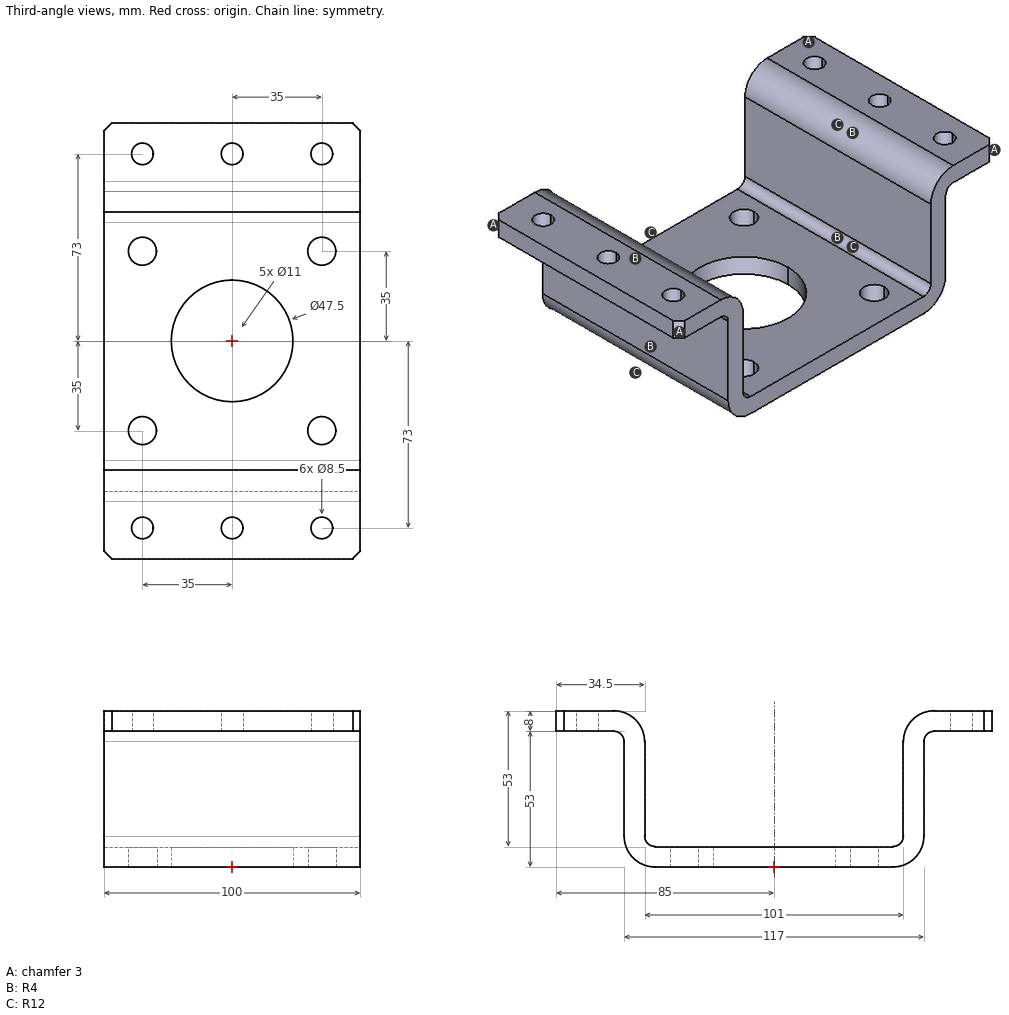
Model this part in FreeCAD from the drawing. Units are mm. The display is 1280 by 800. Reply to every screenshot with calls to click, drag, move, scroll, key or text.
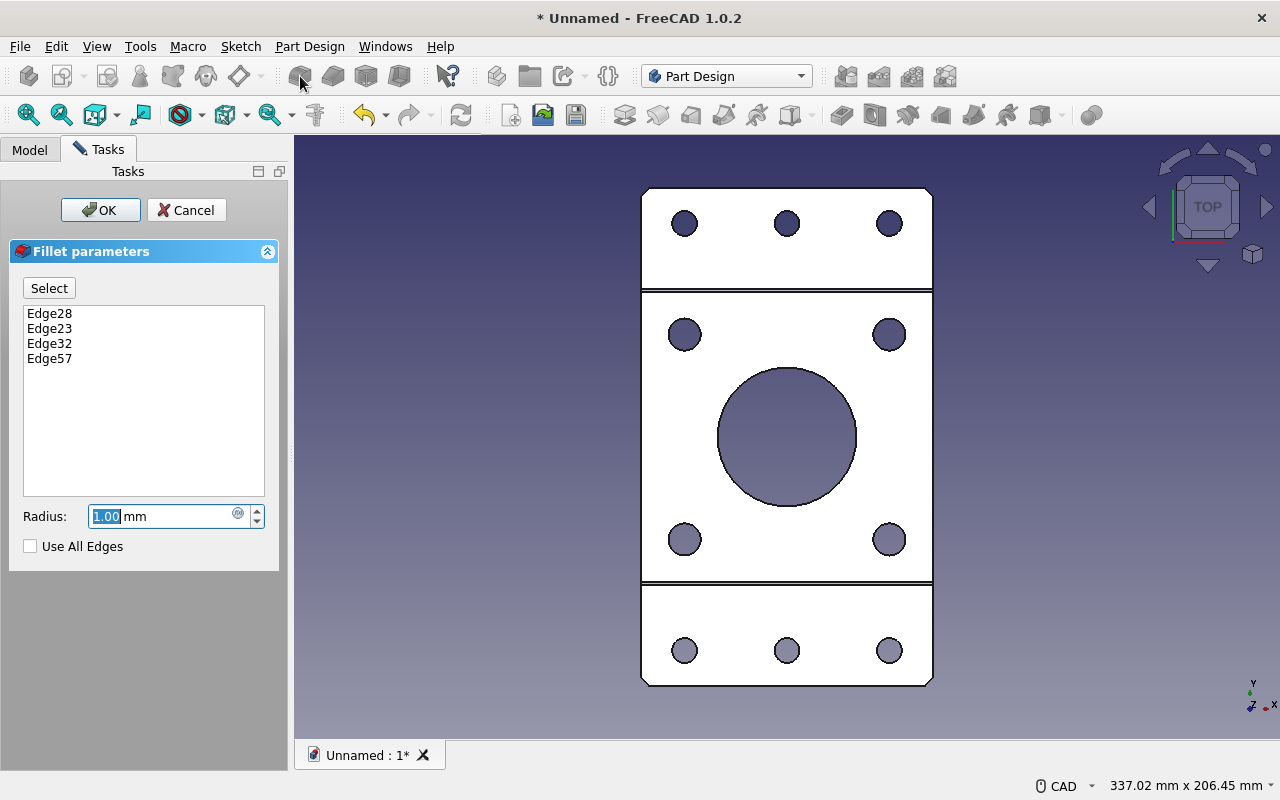
text(4)
key(Tab)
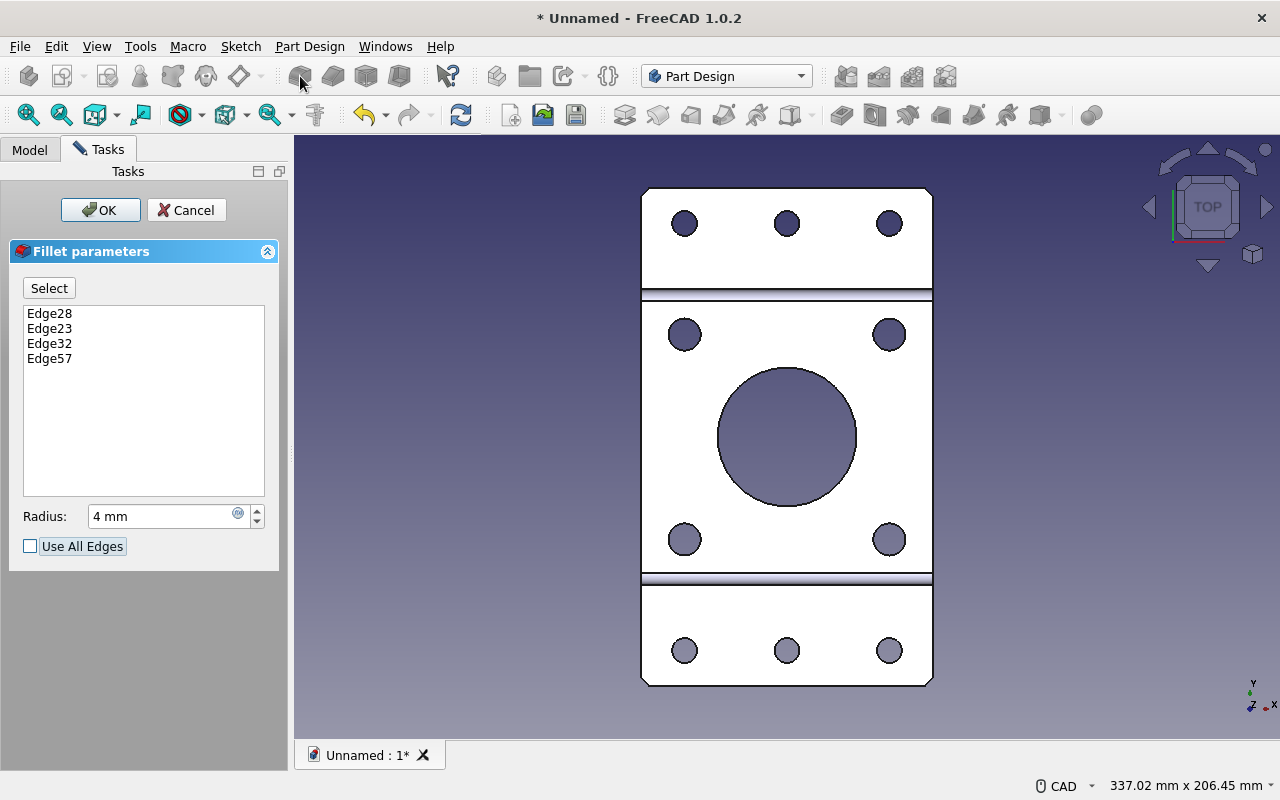
click(101, 210)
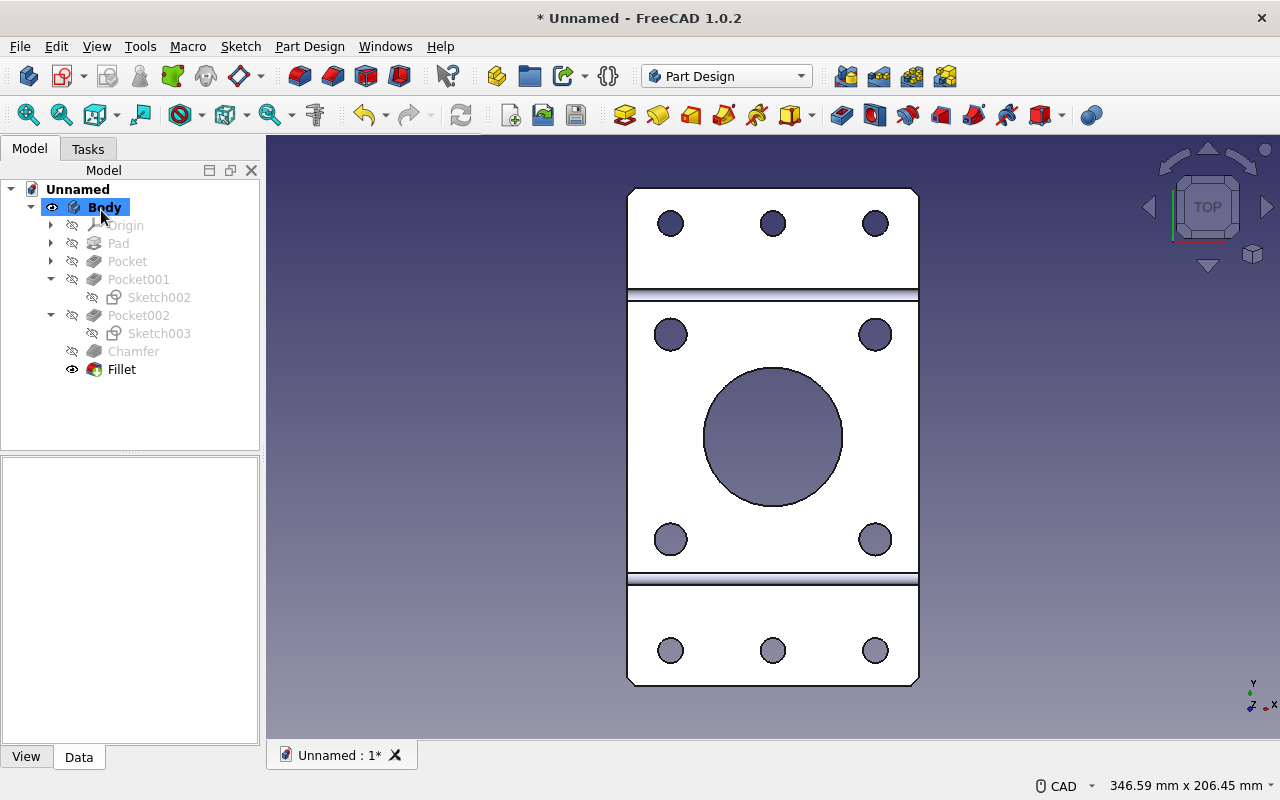
click(773, 584)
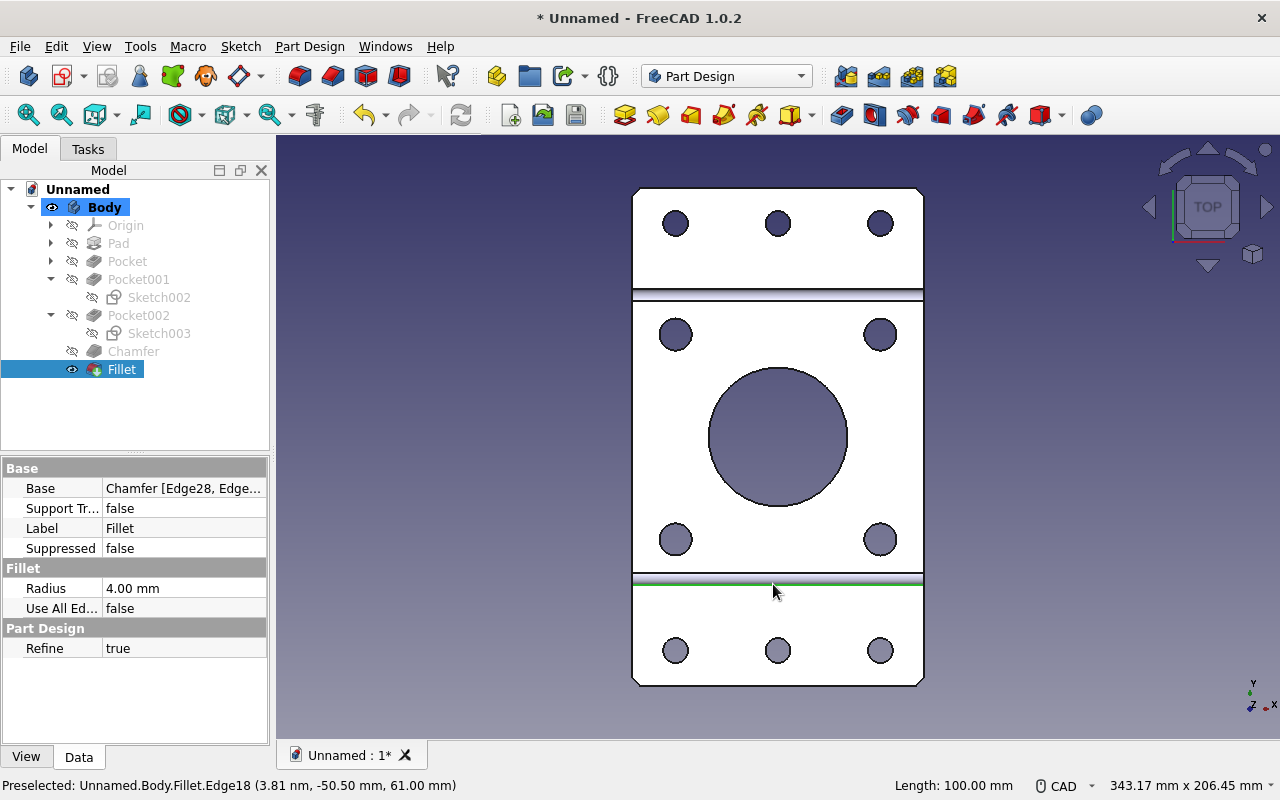
click(778, 288, ctrl)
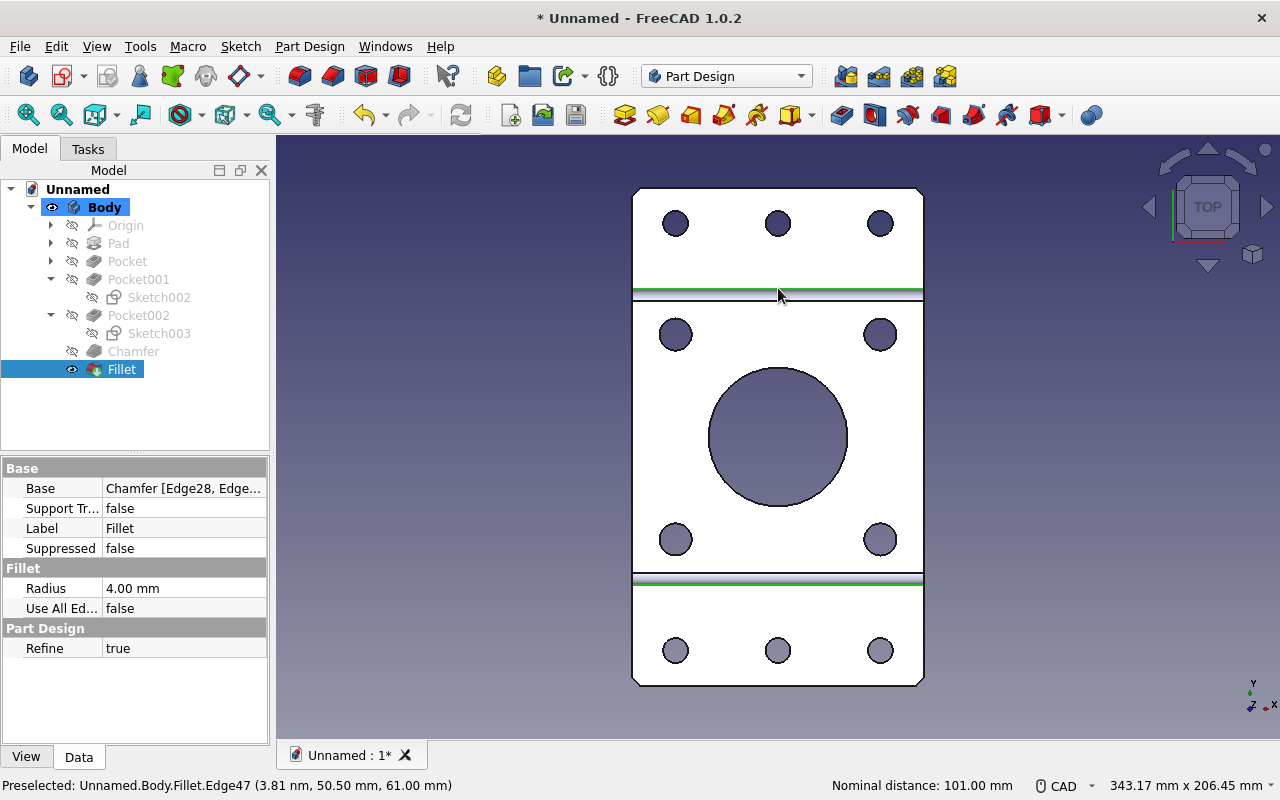
key(0)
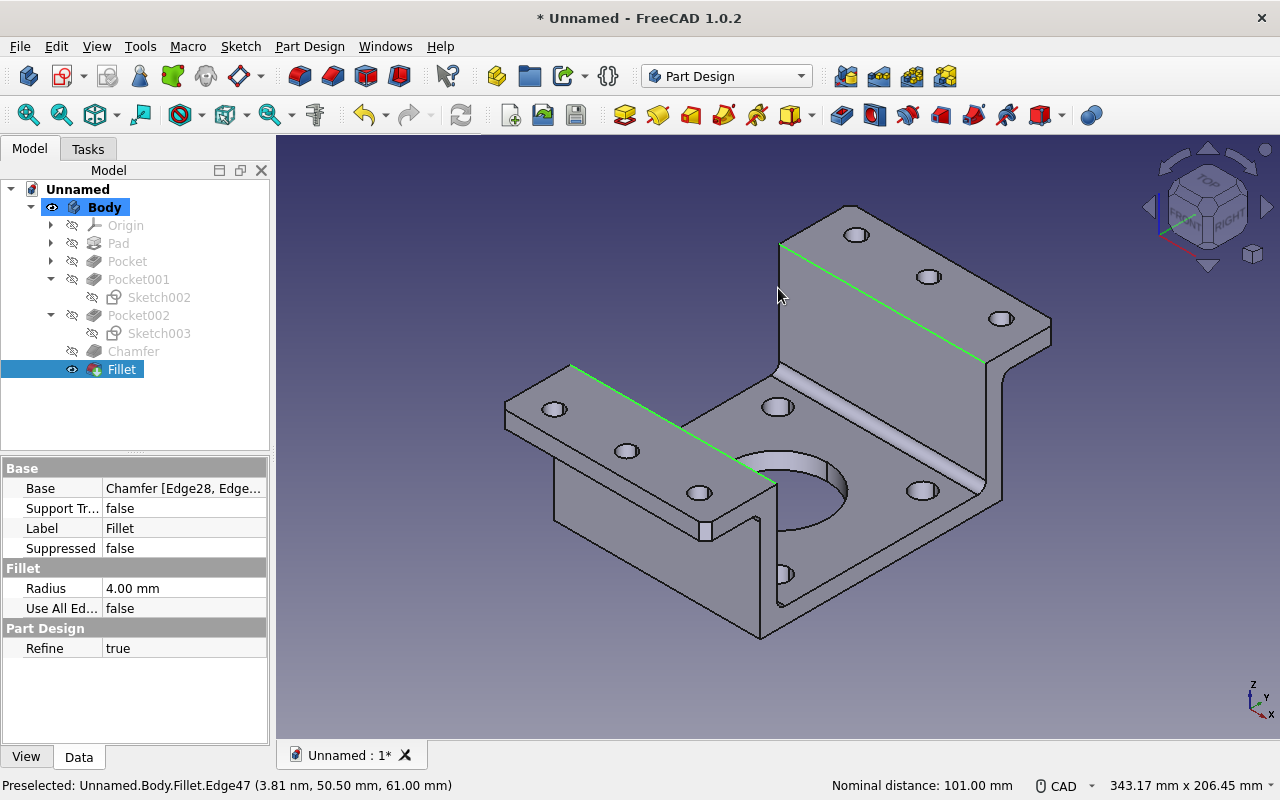
key(2)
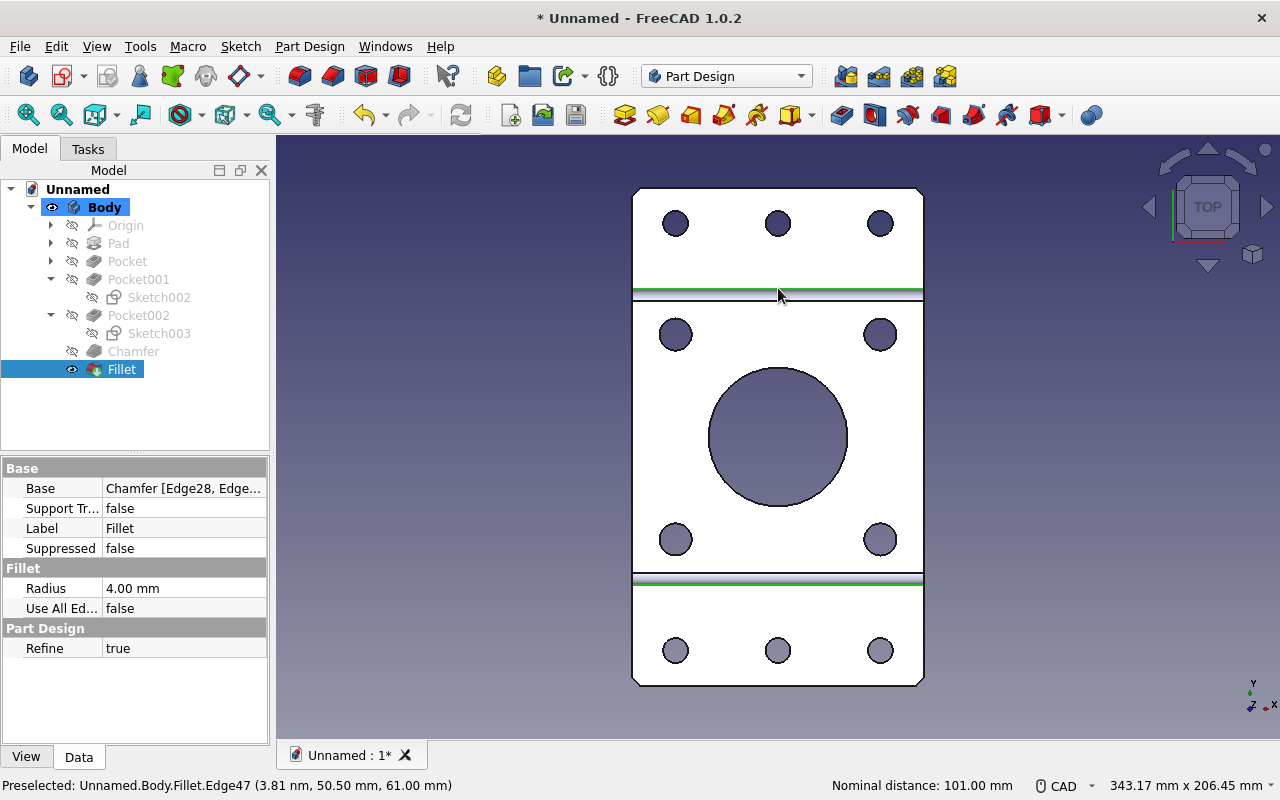
key(1)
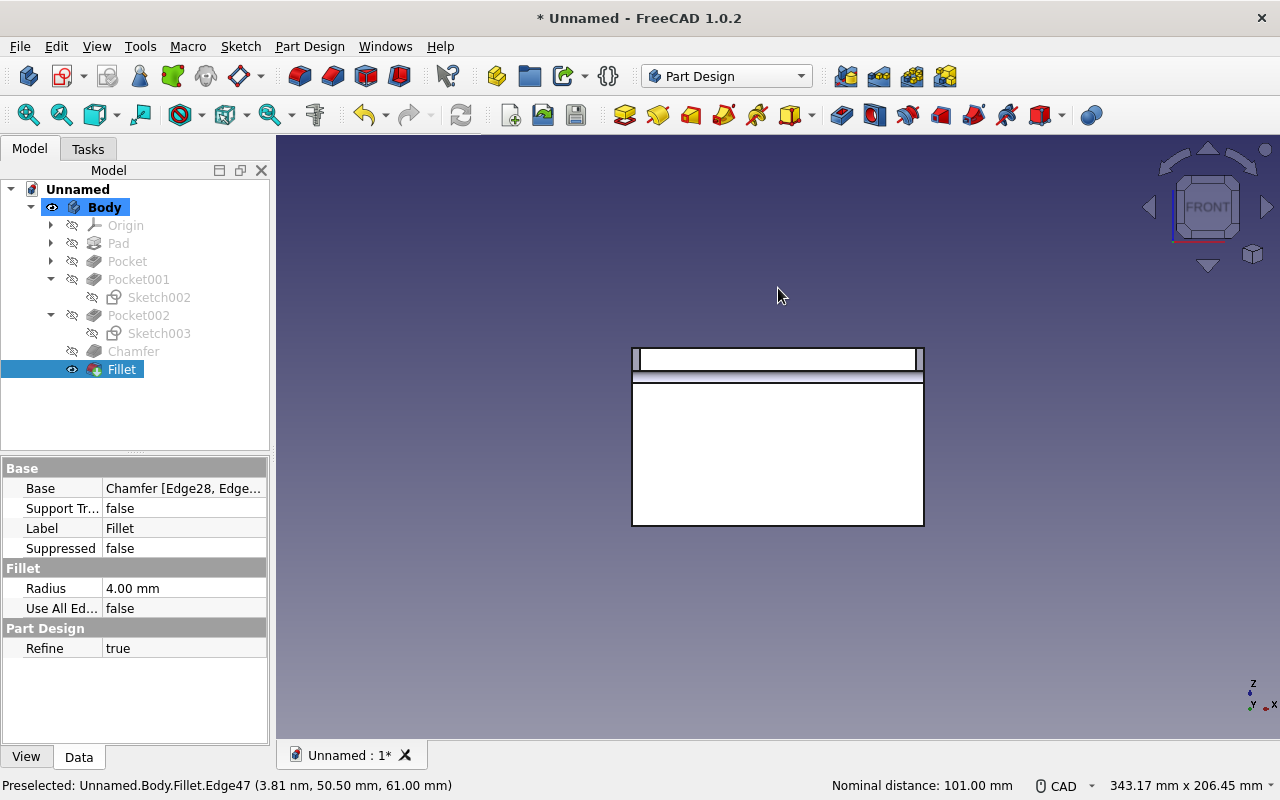
click(29, 116)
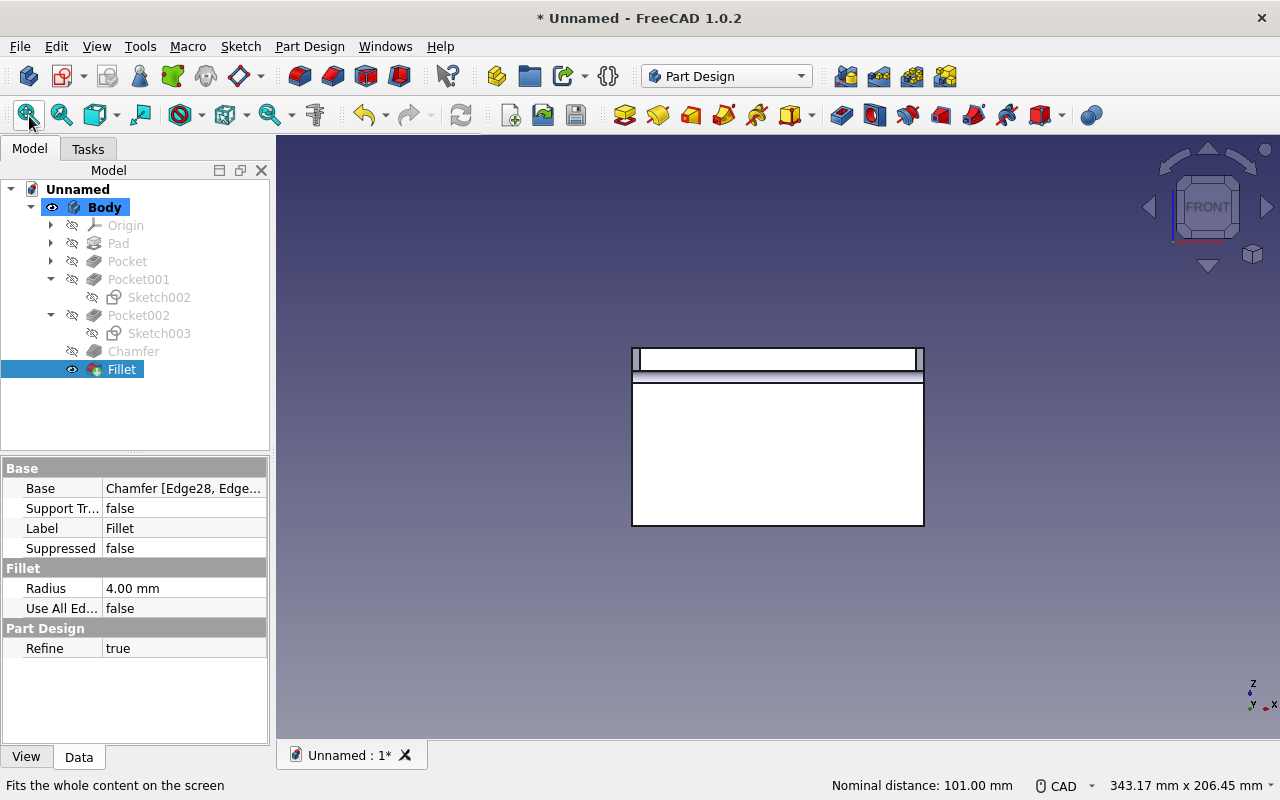
click(778, 525, ctrl)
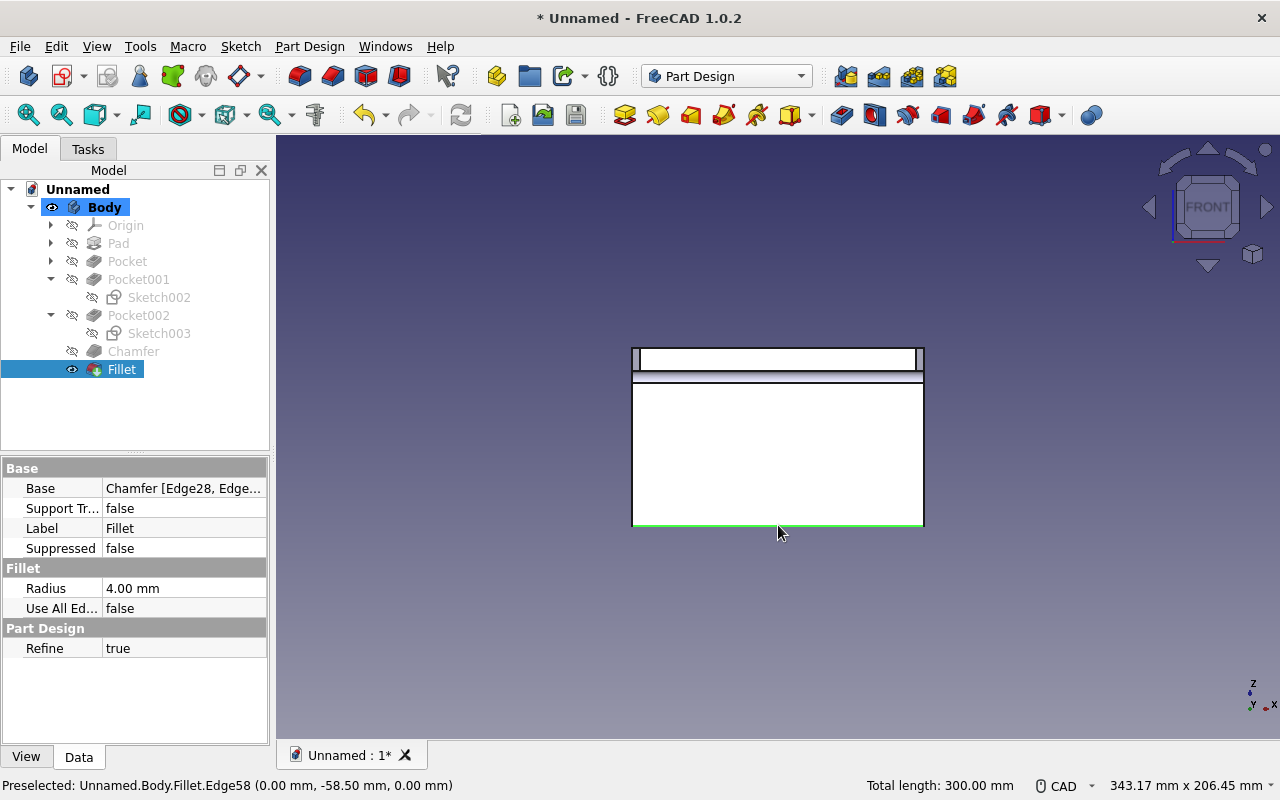
key(3)